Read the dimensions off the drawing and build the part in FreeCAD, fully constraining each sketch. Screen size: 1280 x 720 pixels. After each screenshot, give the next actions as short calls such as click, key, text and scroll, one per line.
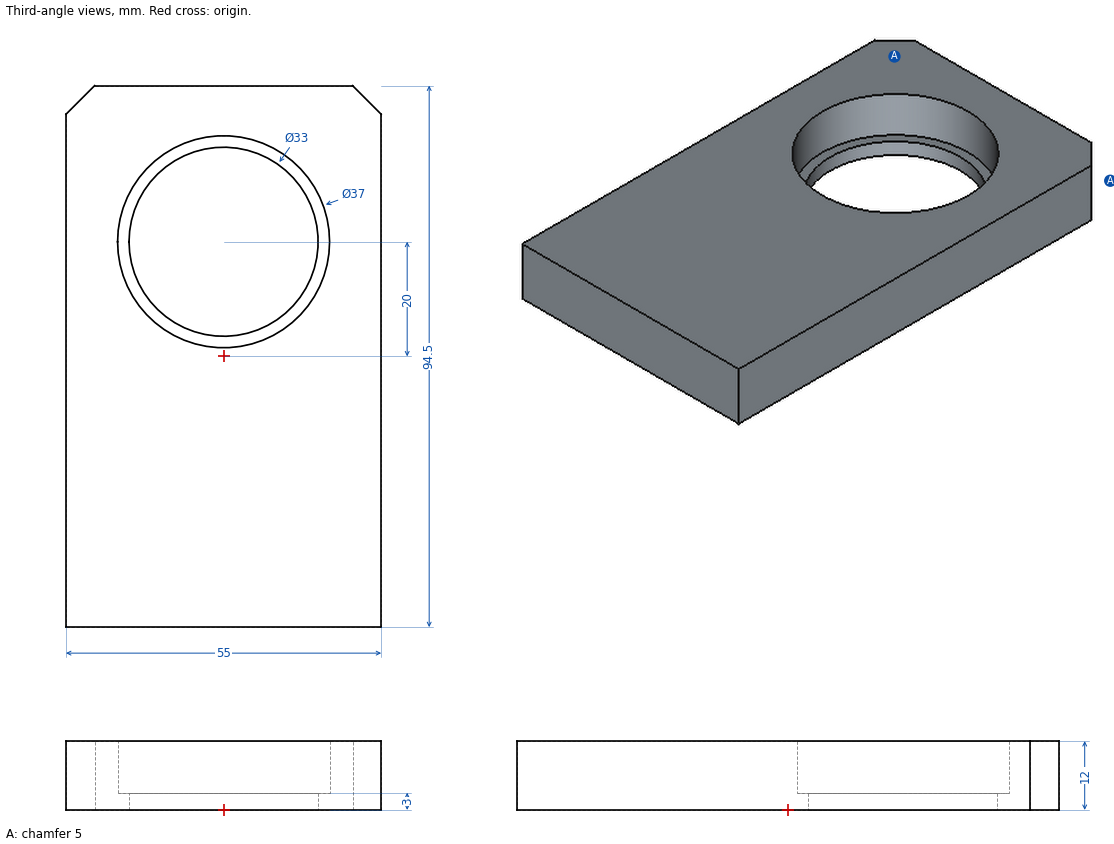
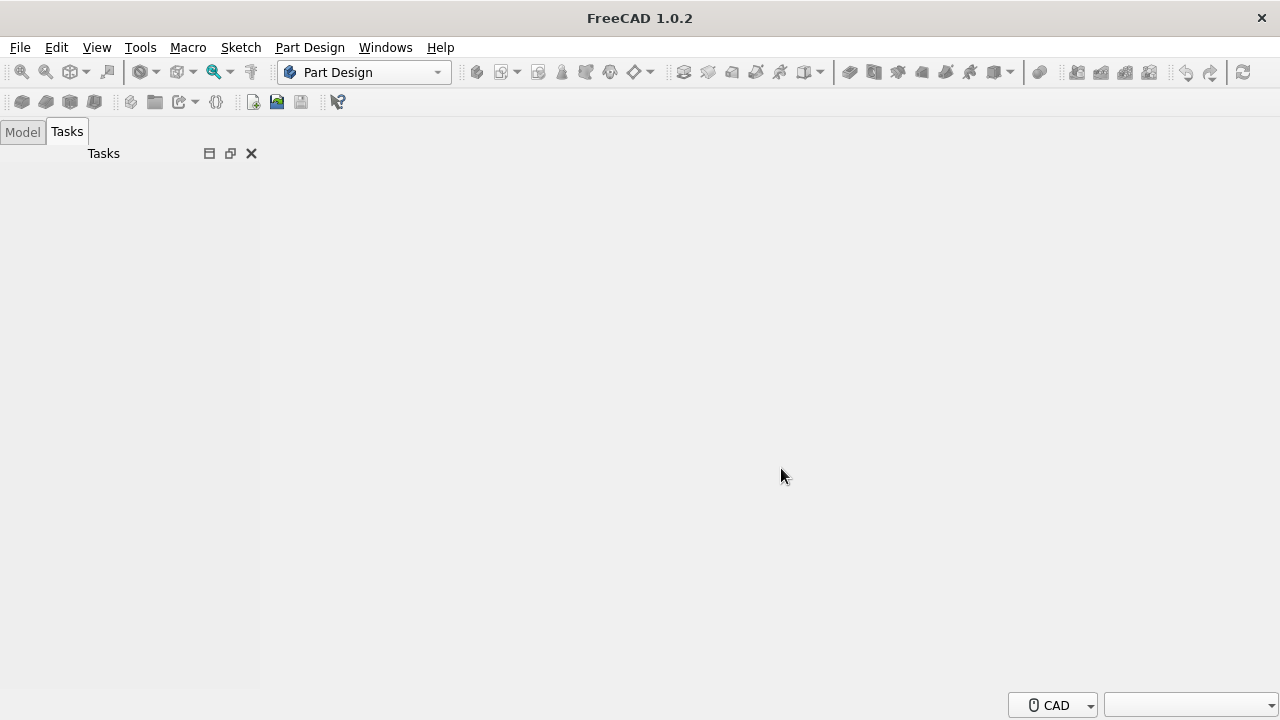
click(254, 102)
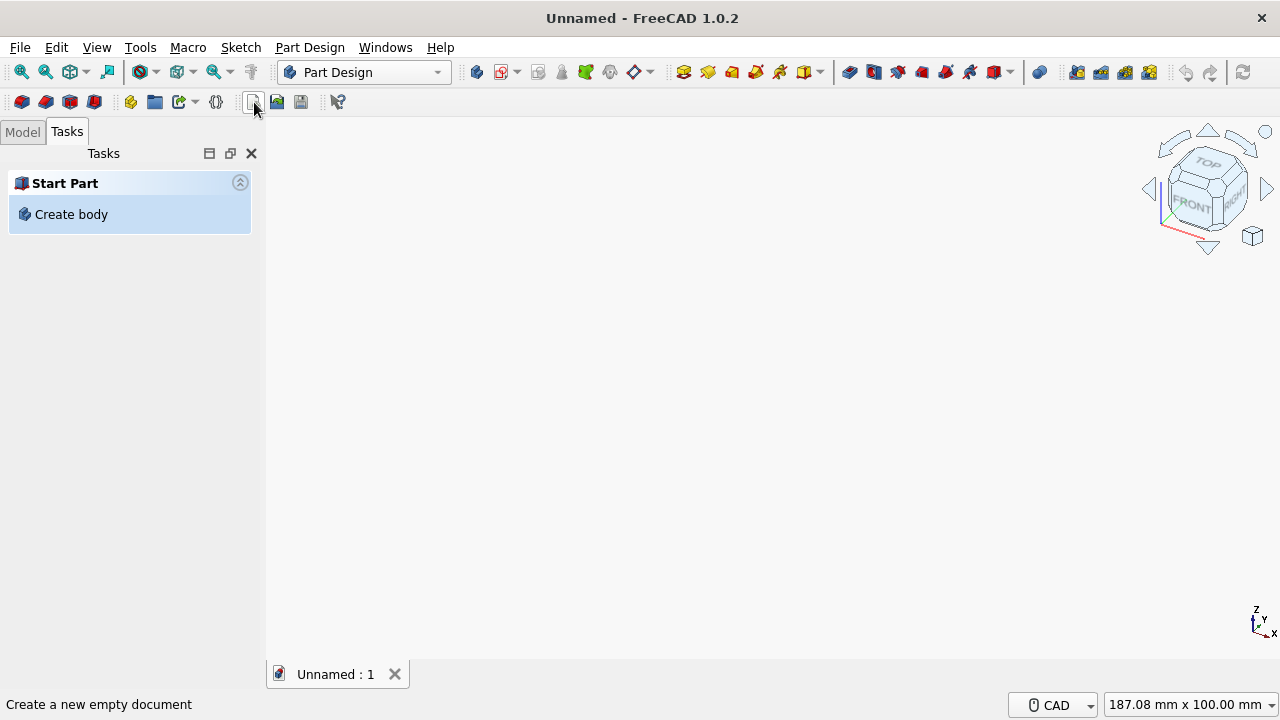
click(502, 72)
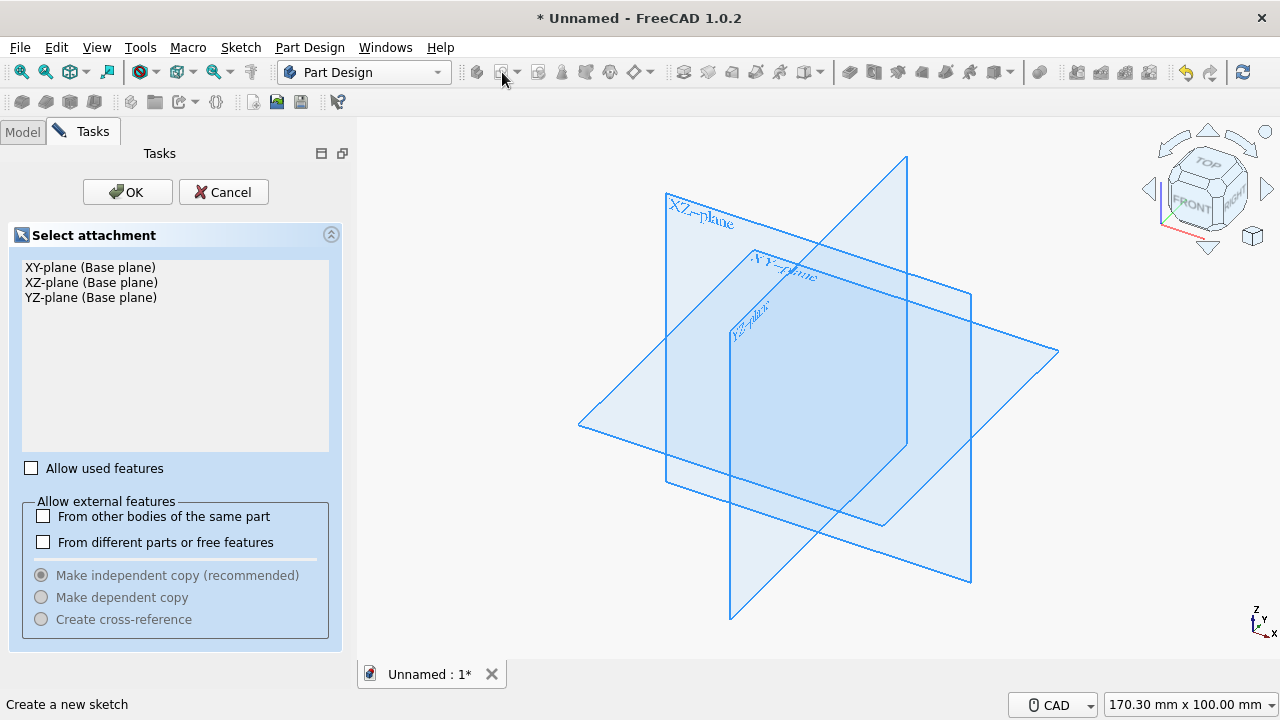
click(82, 268)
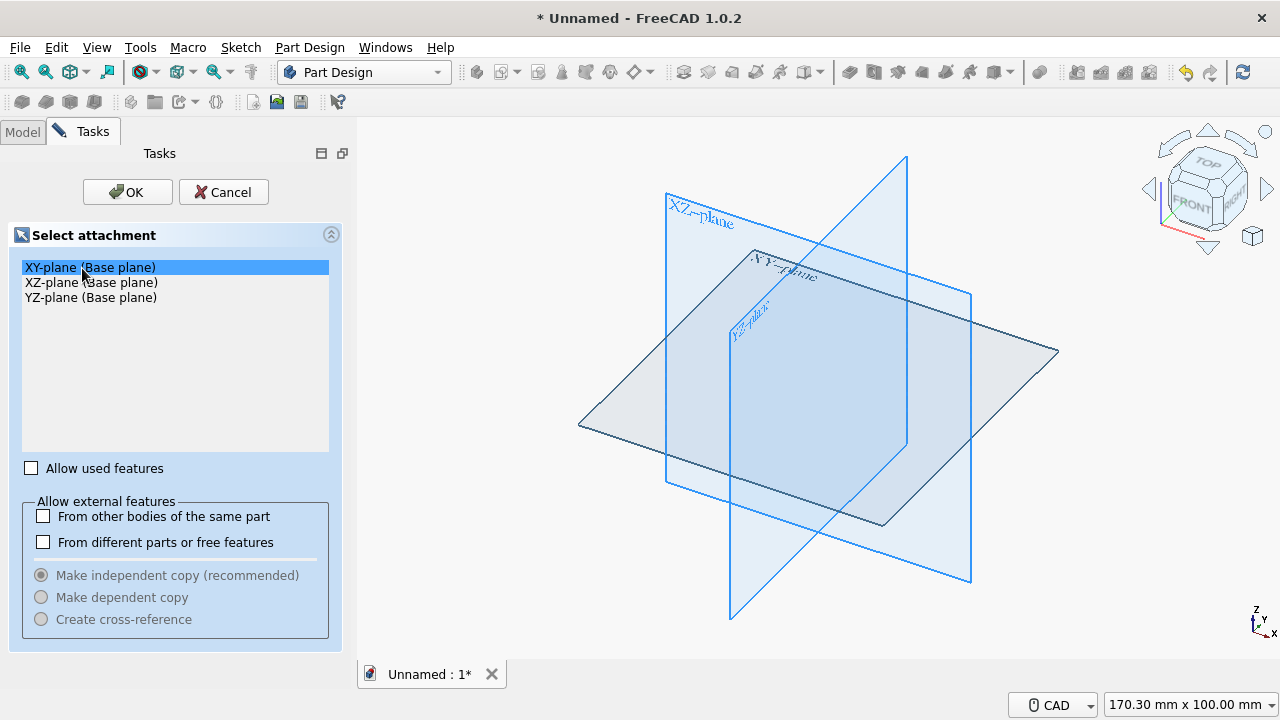
click(128, 192)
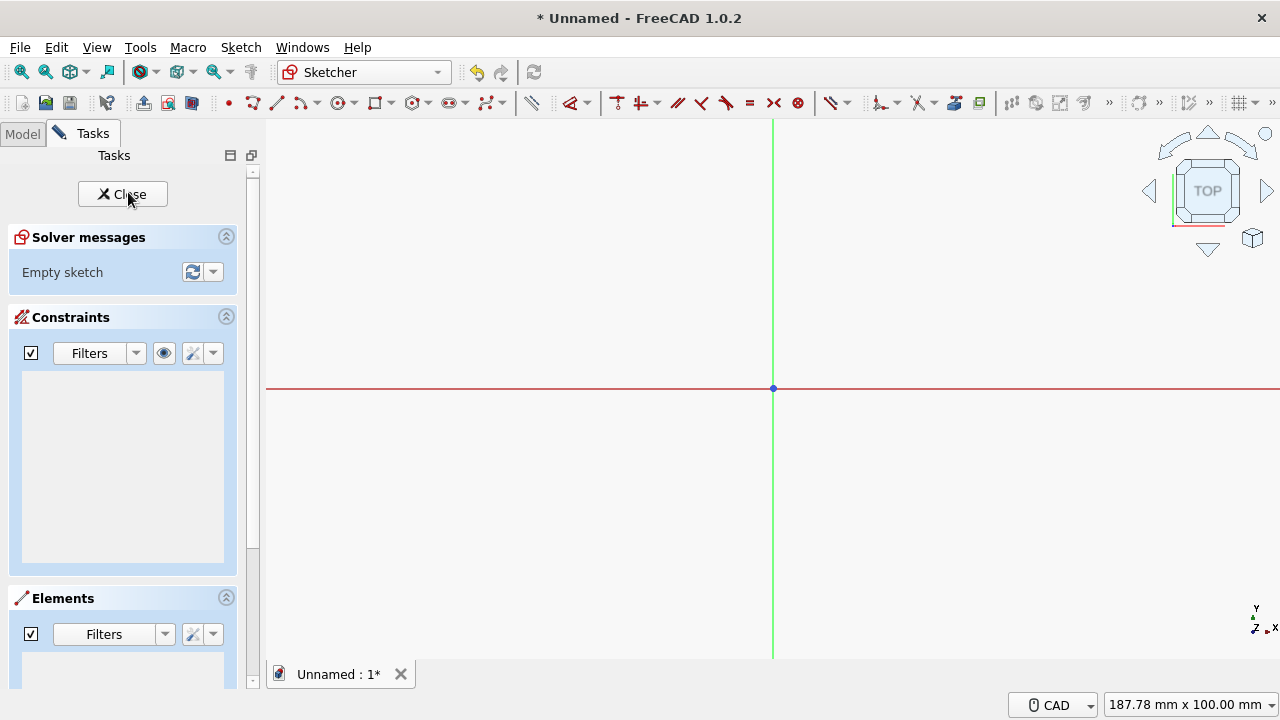
scroll(565, 389, down, 2)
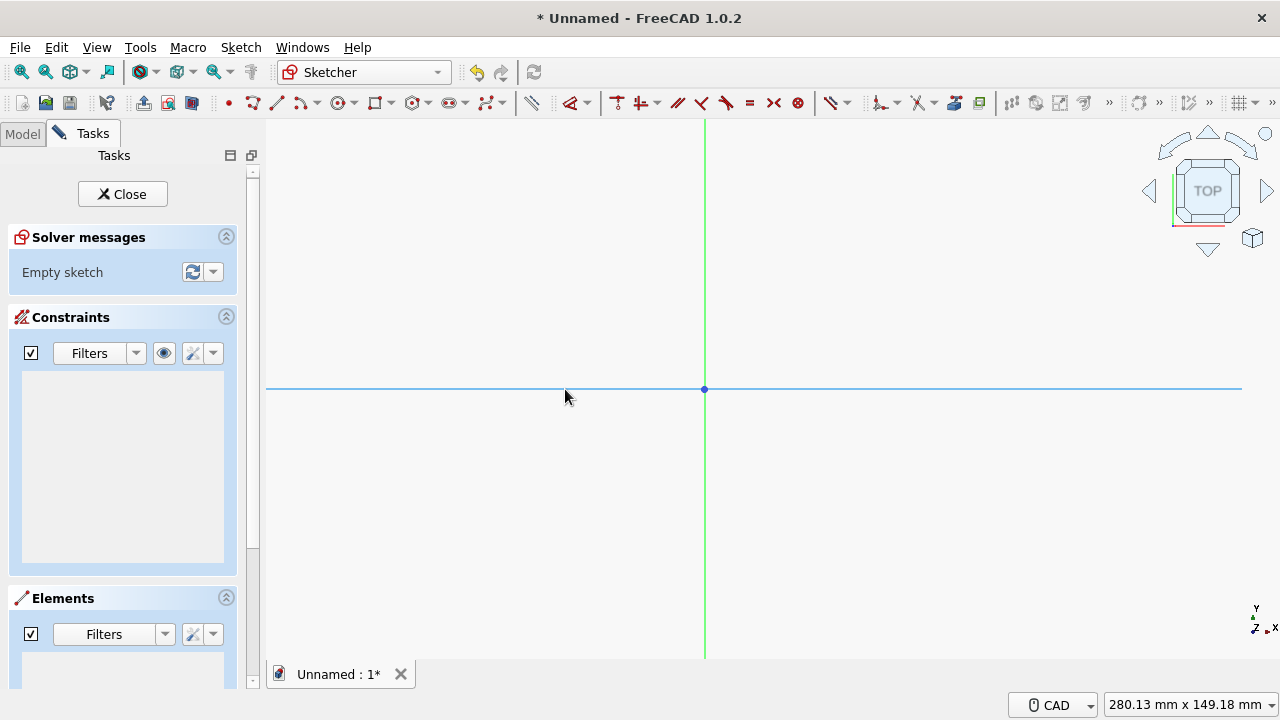
key(g)
key(v)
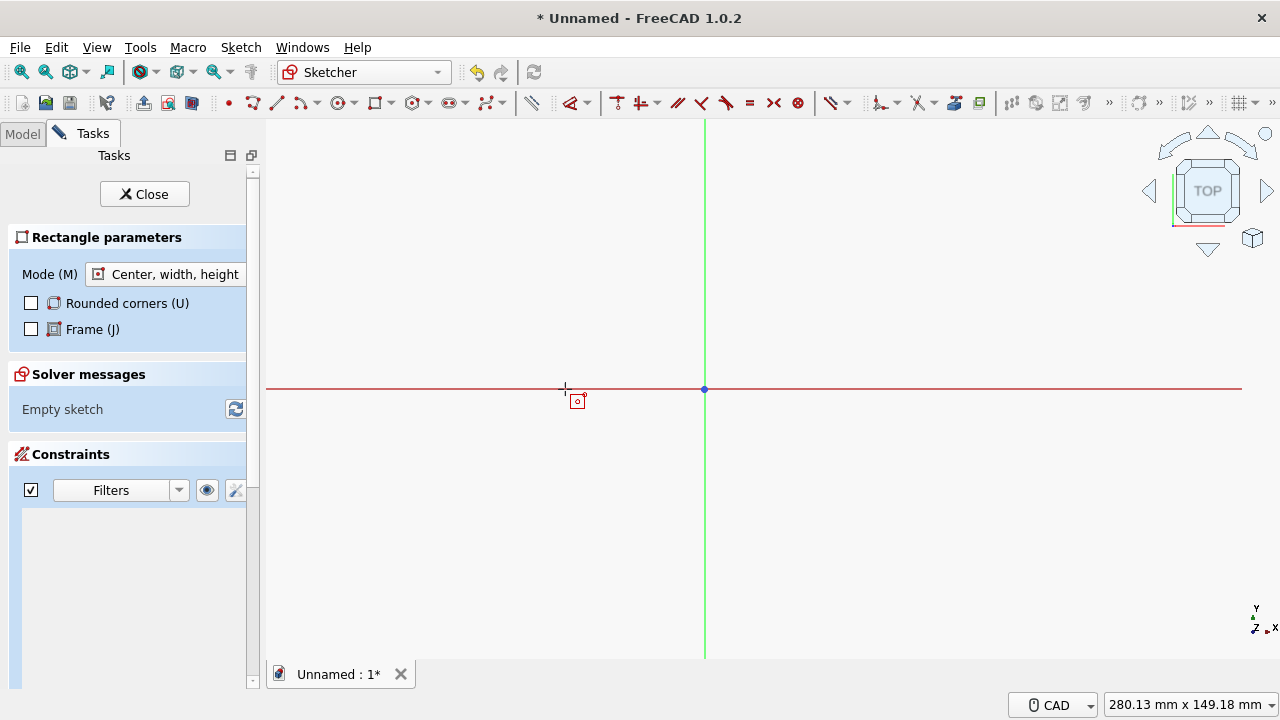
click(705, 389)
click(804, 218)
key(Escape)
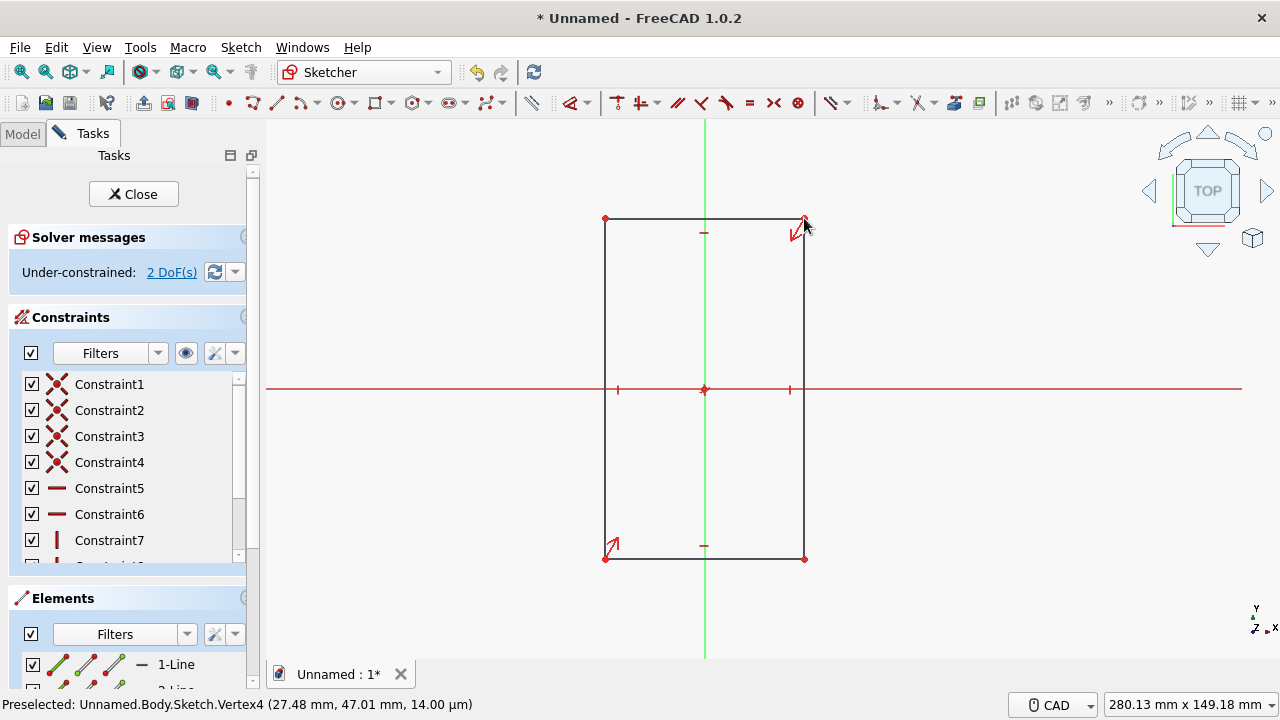
click(665, 559)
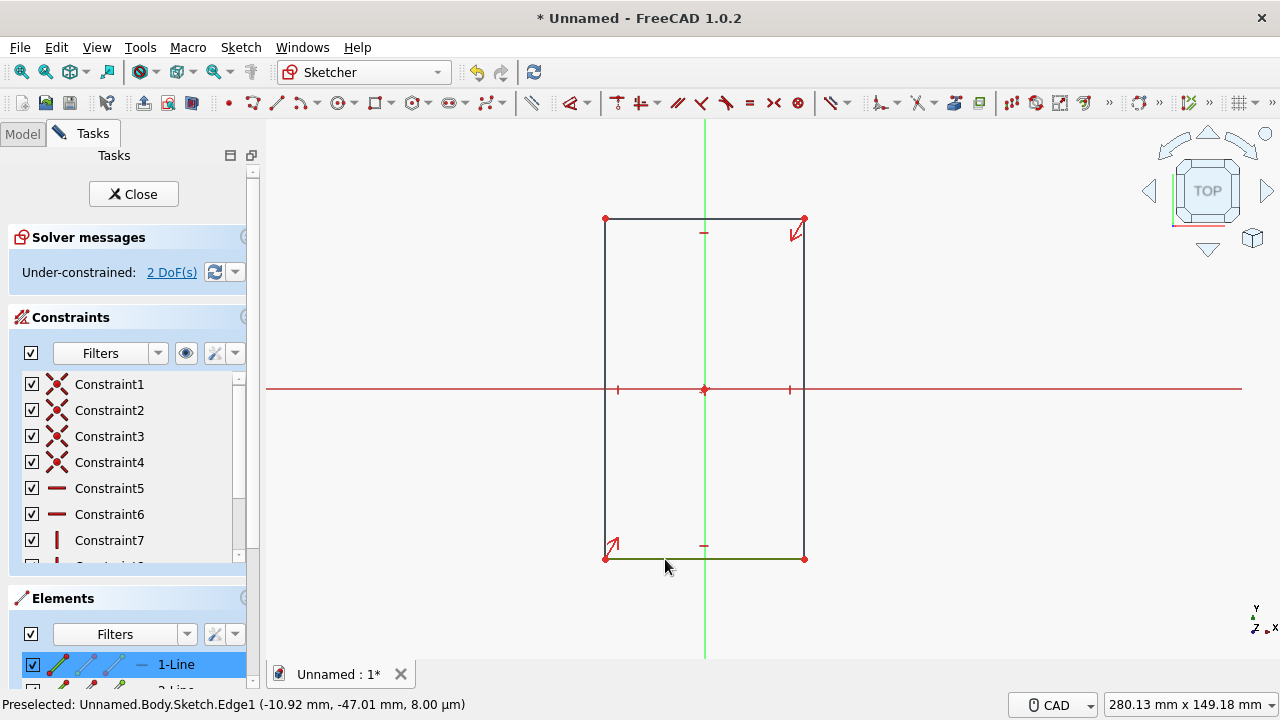
click(590, 104)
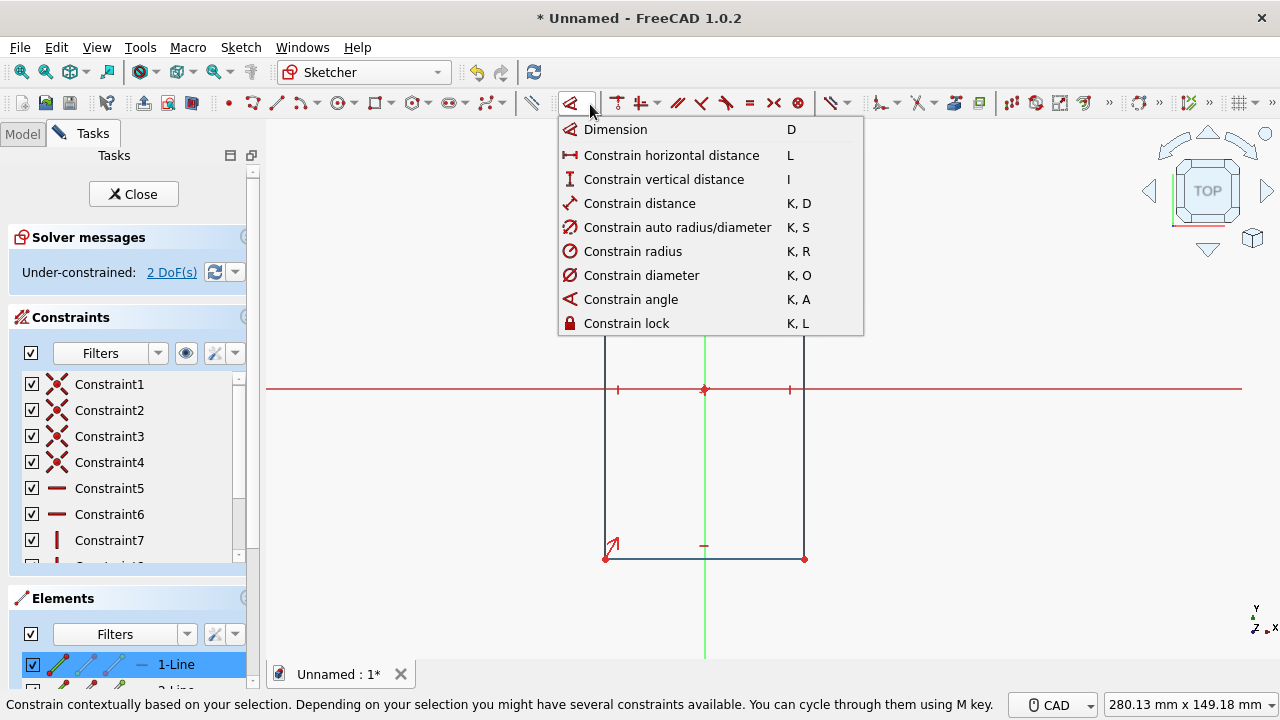
click(711, 155)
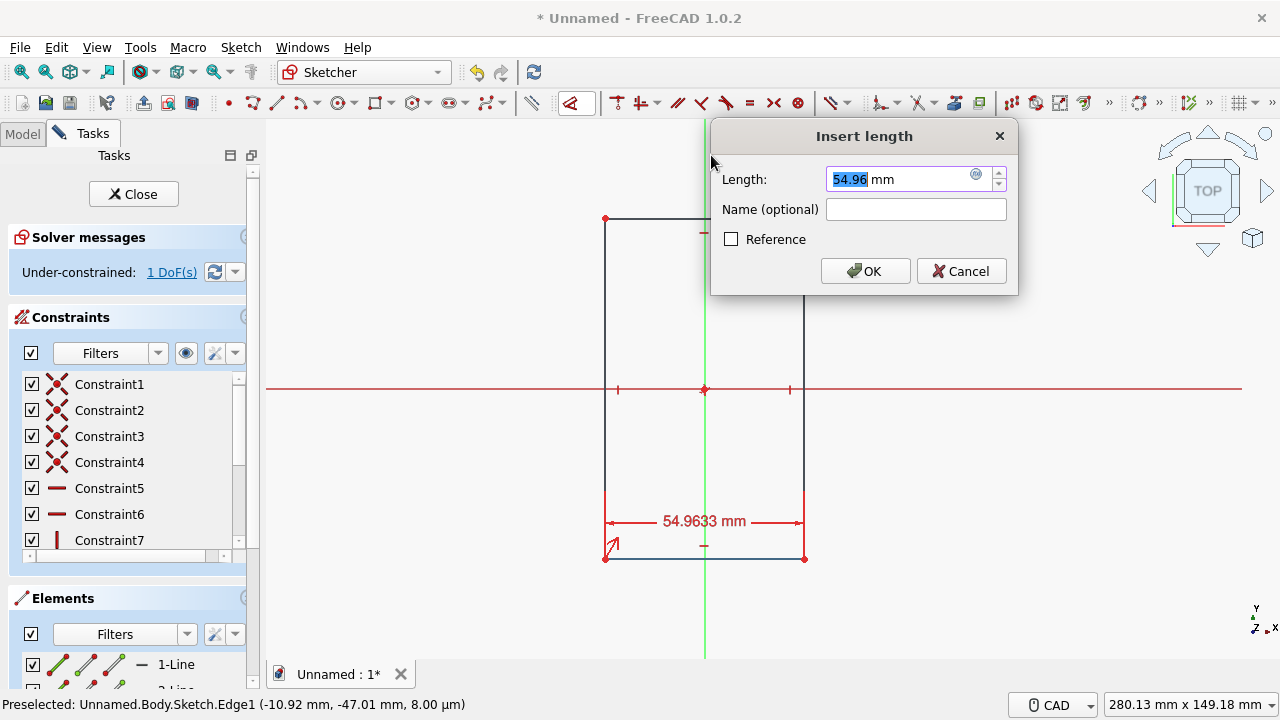
text(55)
key(Return)